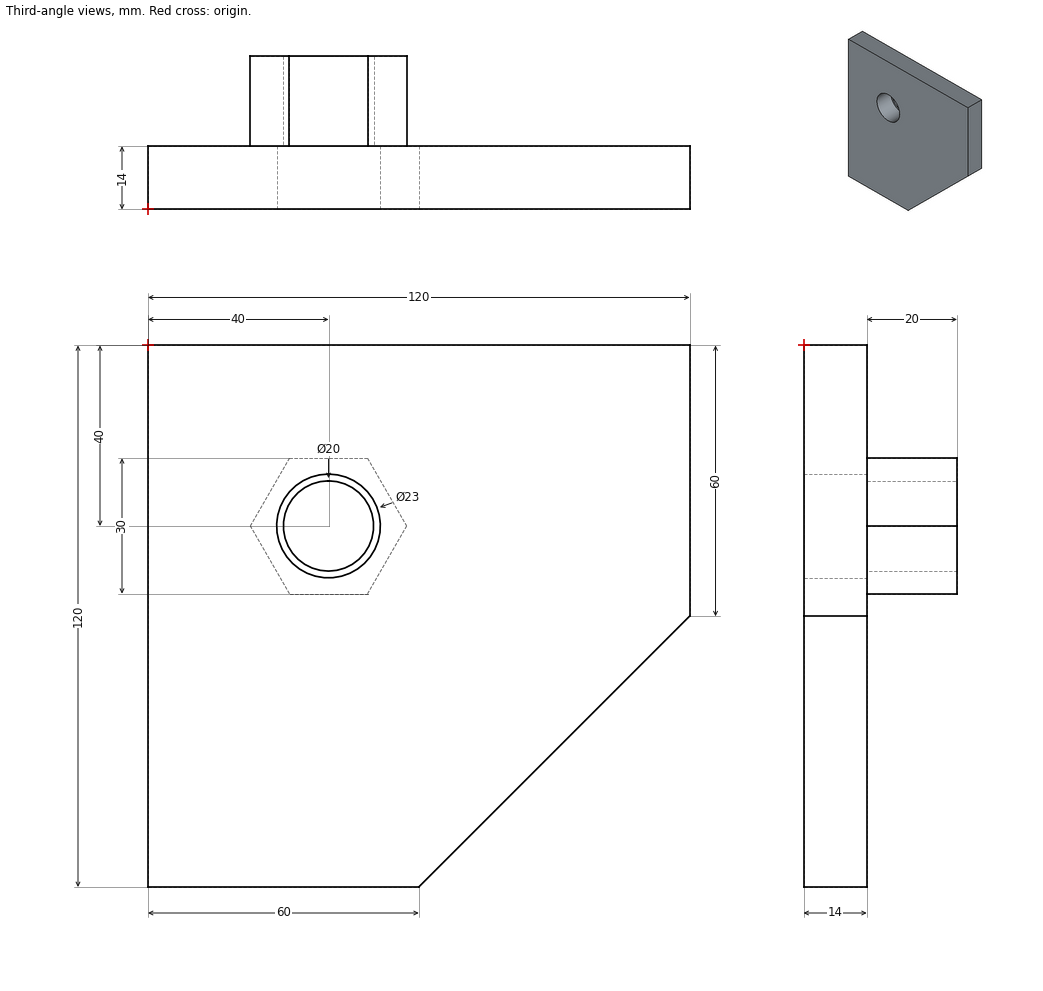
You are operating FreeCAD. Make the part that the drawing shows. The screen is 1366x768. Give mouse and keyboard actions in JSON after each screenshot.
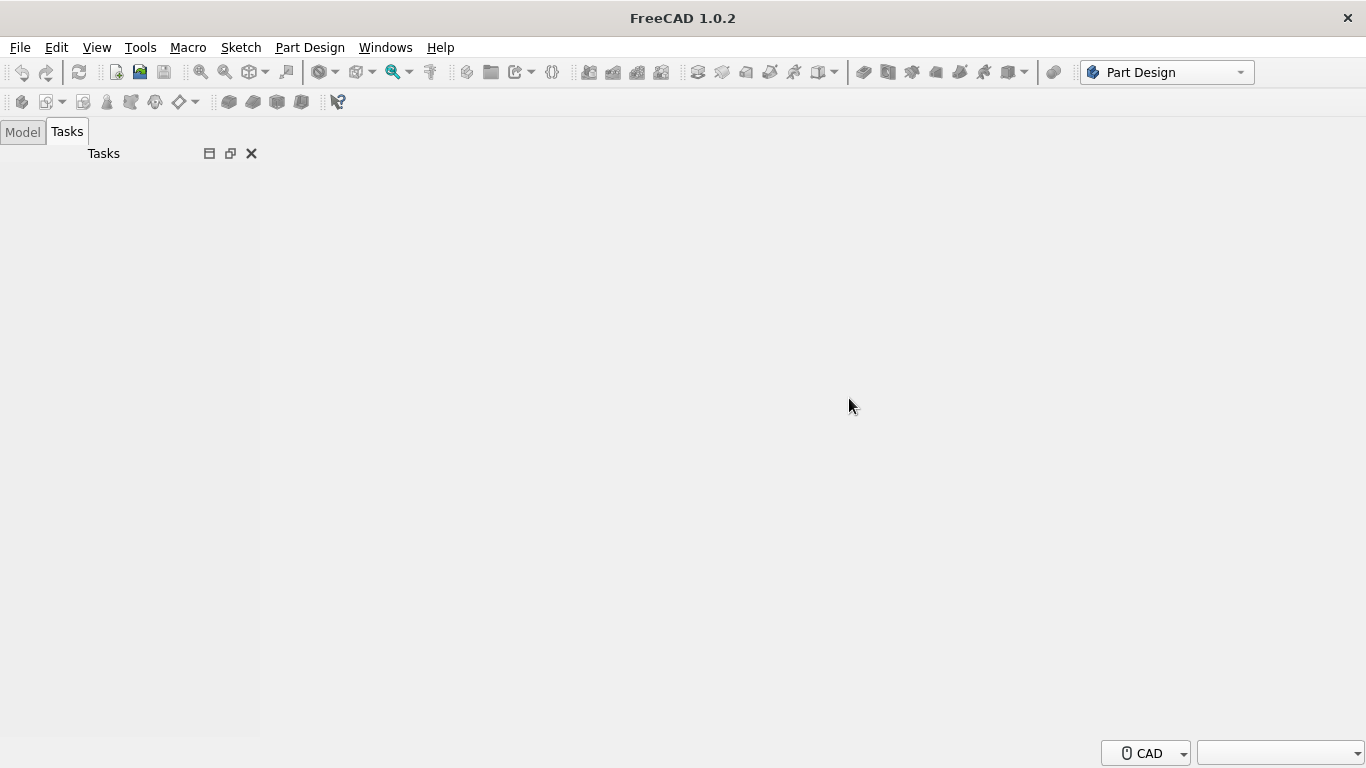
{"action": "left_click", "coordinate": [116, 72]}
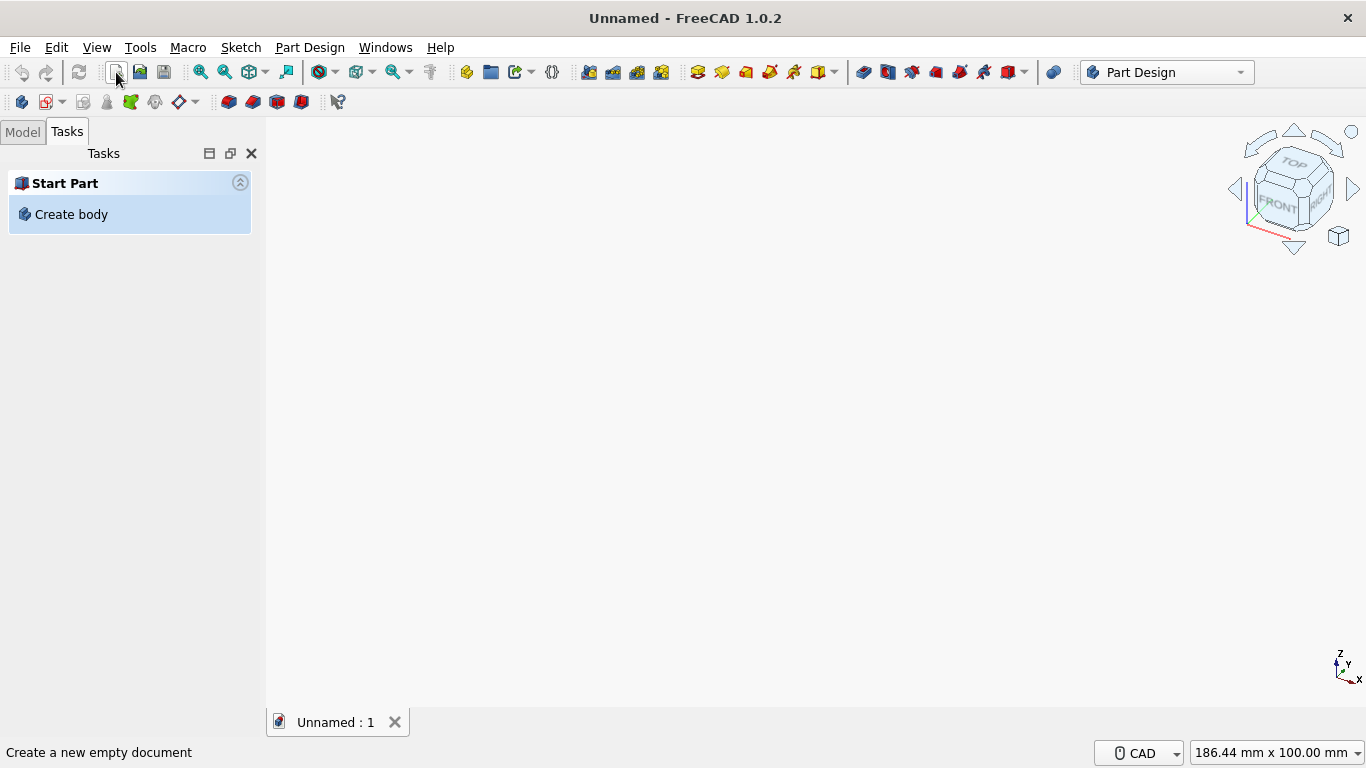
{"action": "left_click", "coordinate": [46, 102]}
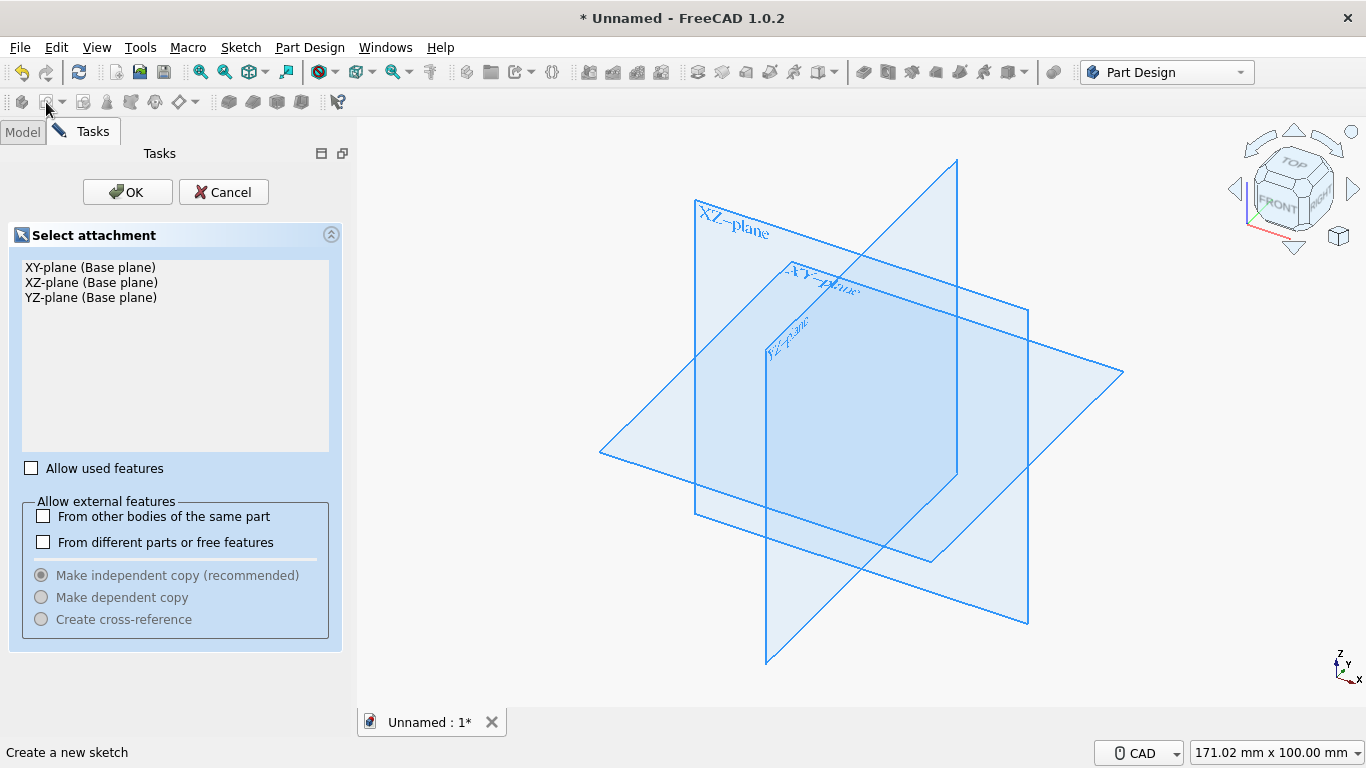
{"action": "left_click", "coordinate": [82, 282]}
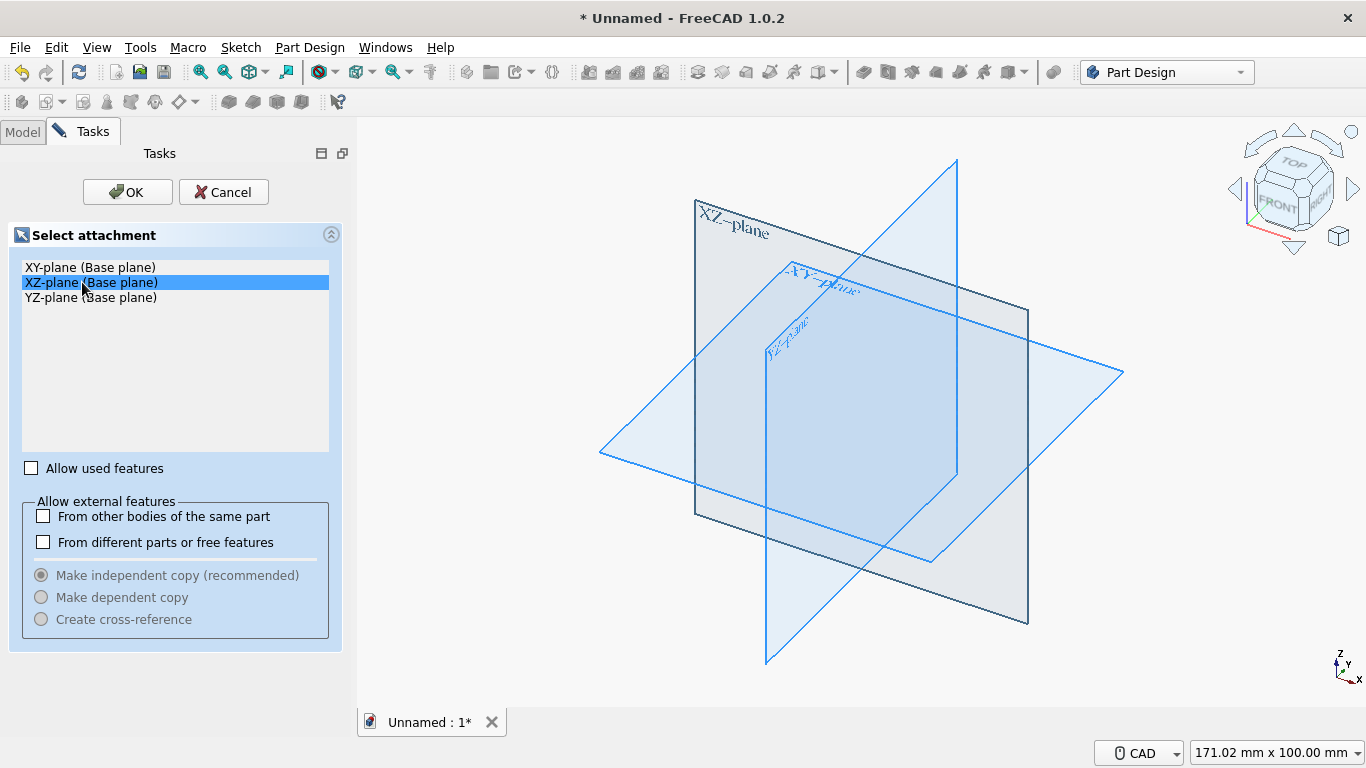
{"action": "left_click", "coordinate": [128, 192]}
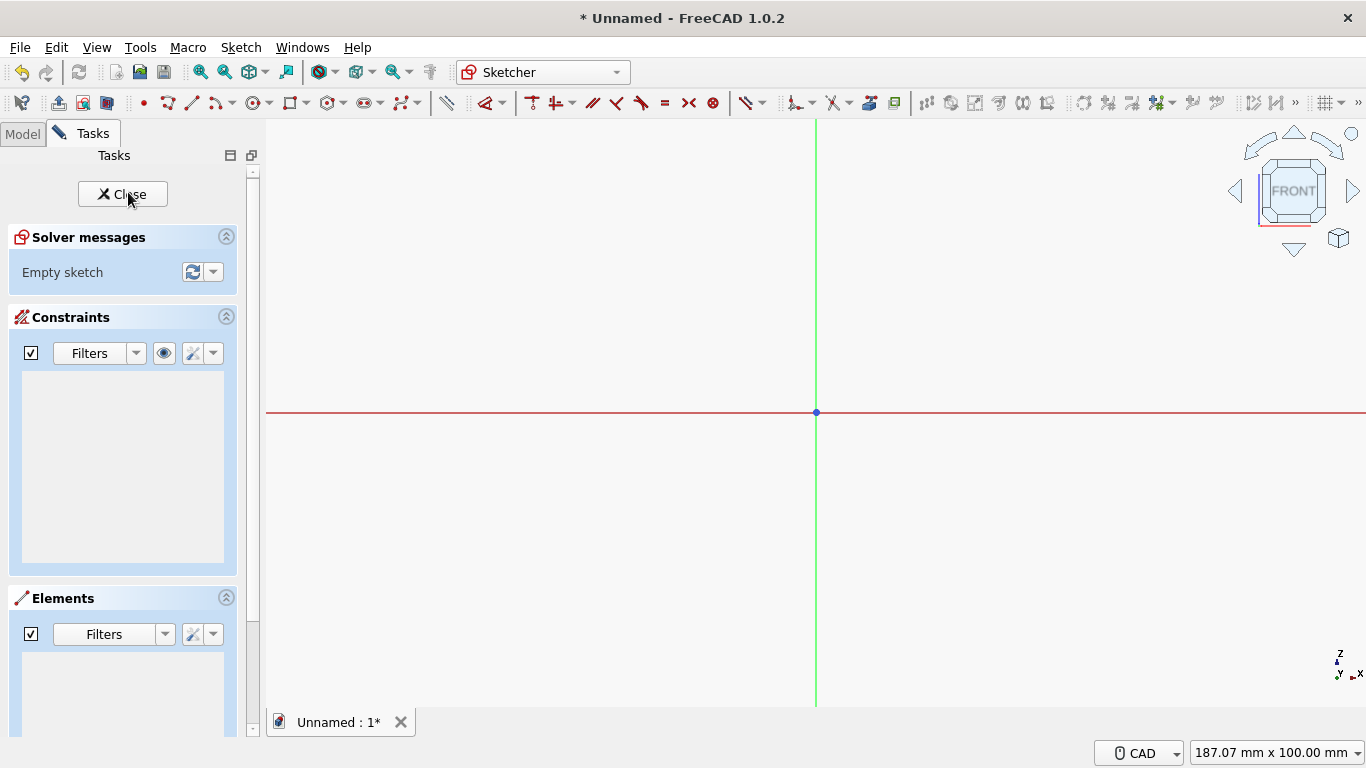
{"action": "scroll", "coordinate": [404, 147], "scroll_direction": "down", "scroll_amount": 4}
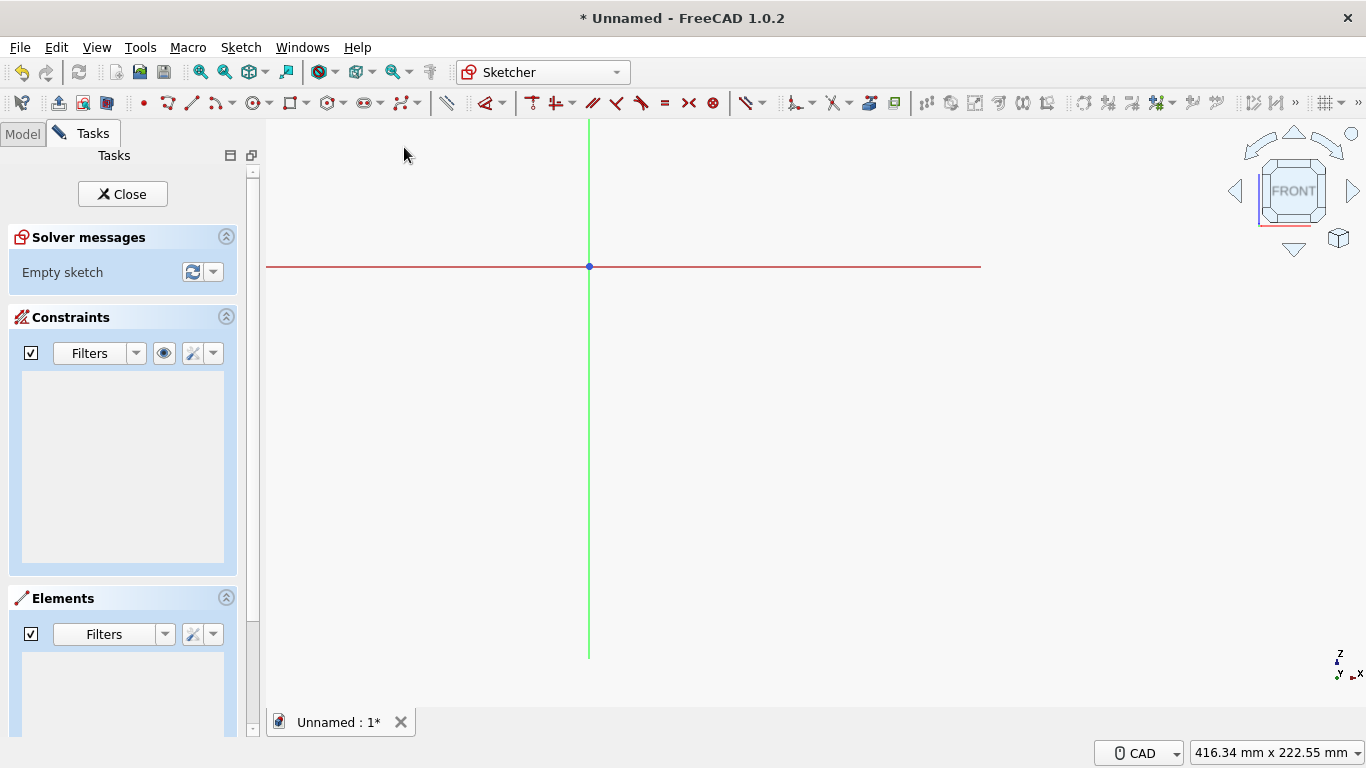
{"action": "left_click", "coordinate": [168, 104]}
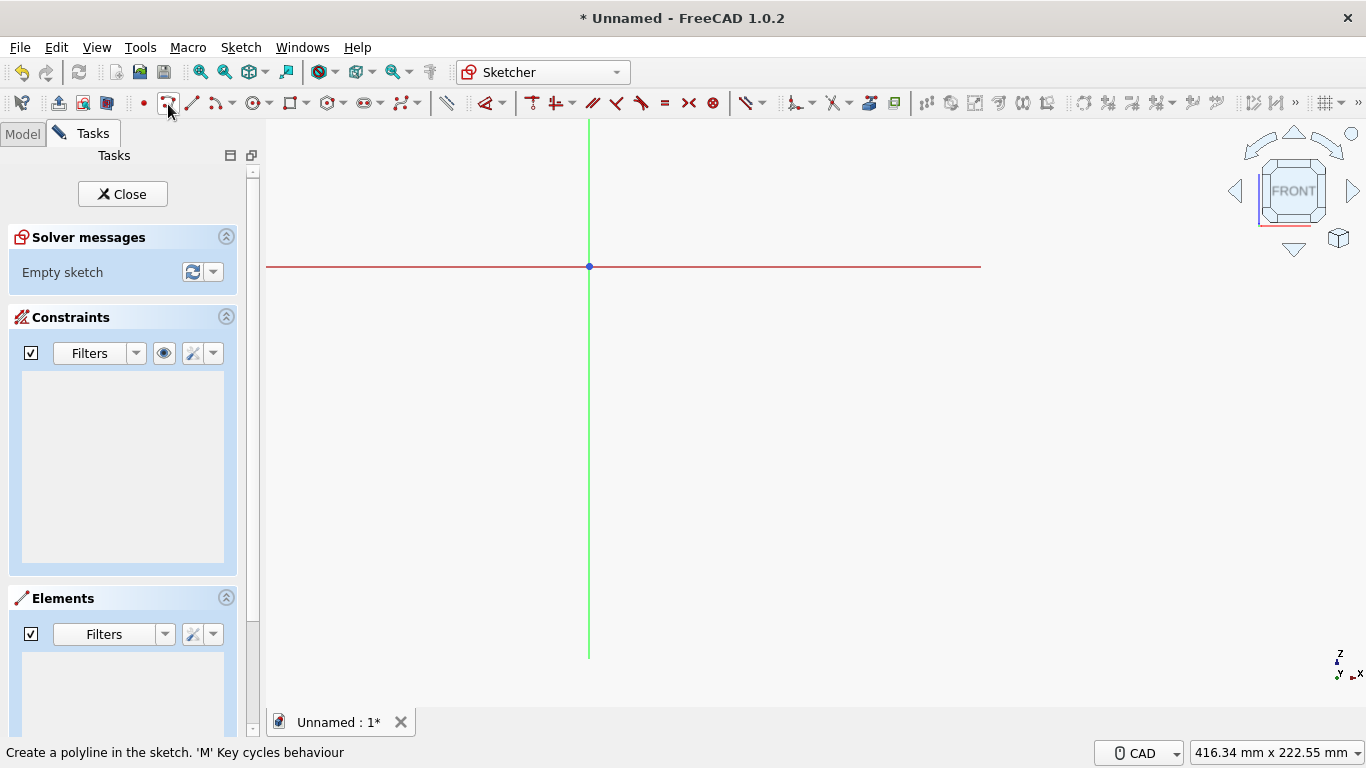
{"action": "left_click", "coordinate": [589, 267]}
{"action": "left_click", "coordinate": [906, 276]}
{"action": "left_click", "coordinate": [906, 425]}
{"action": "left_click", "coordinate": [748, 584]}
{"action": "left_click", "coordinate": [598, 584]}
{"action": "left_click", "coordinate": [589, 267]}
{"action": "key", "text": "Escape"}
{"action": "key", "text": "Escape"}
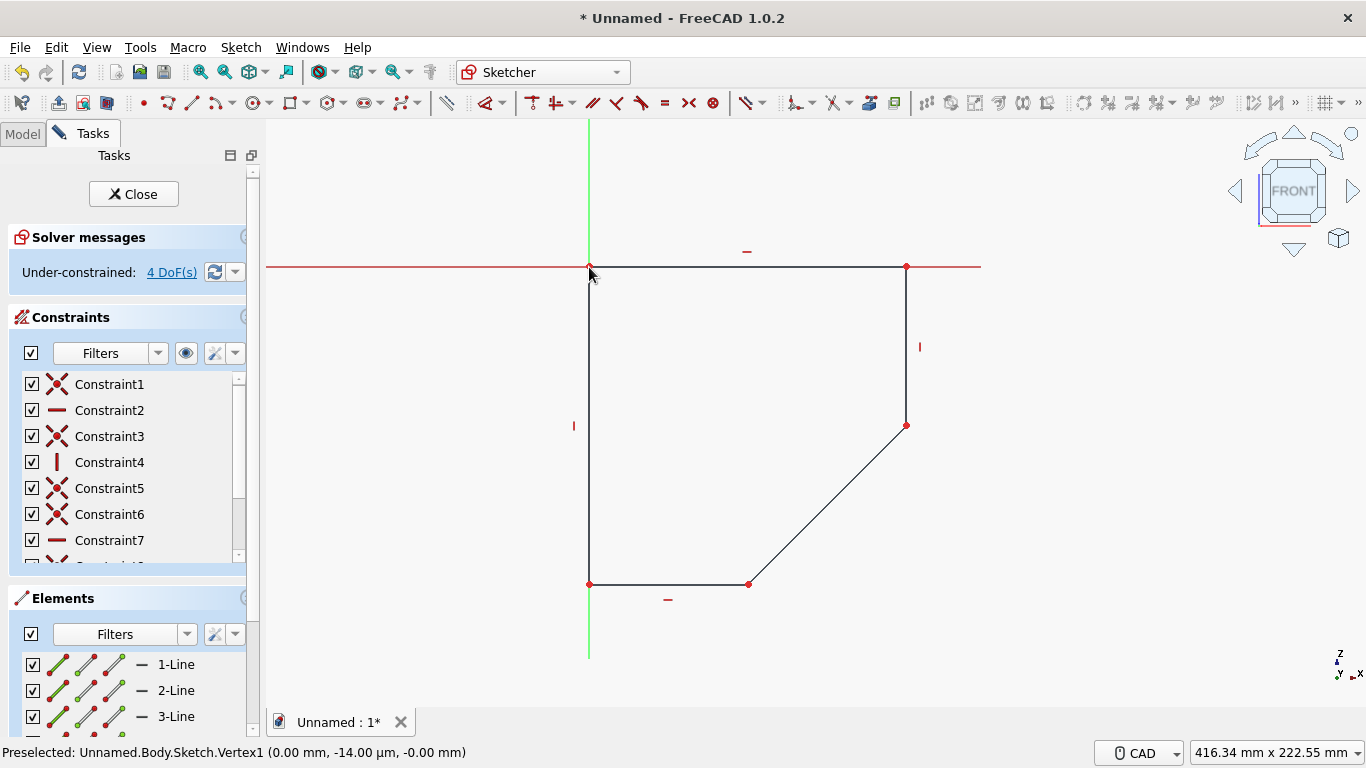
{"action": "left_click", "coordinate": [486, 104]}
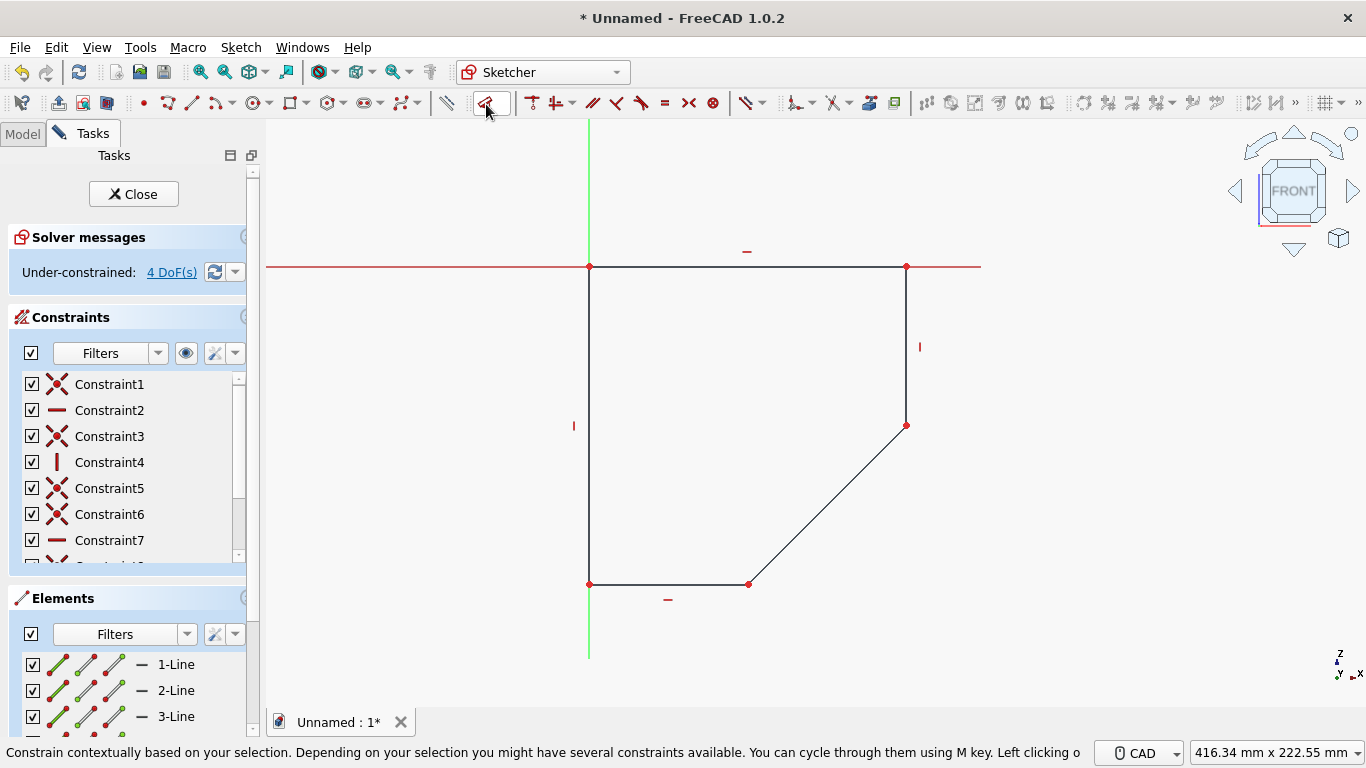
{"action": "left_click", "coordinate": [906, 314]}
{"action": "left_click", "coordinate": [940, 346]}